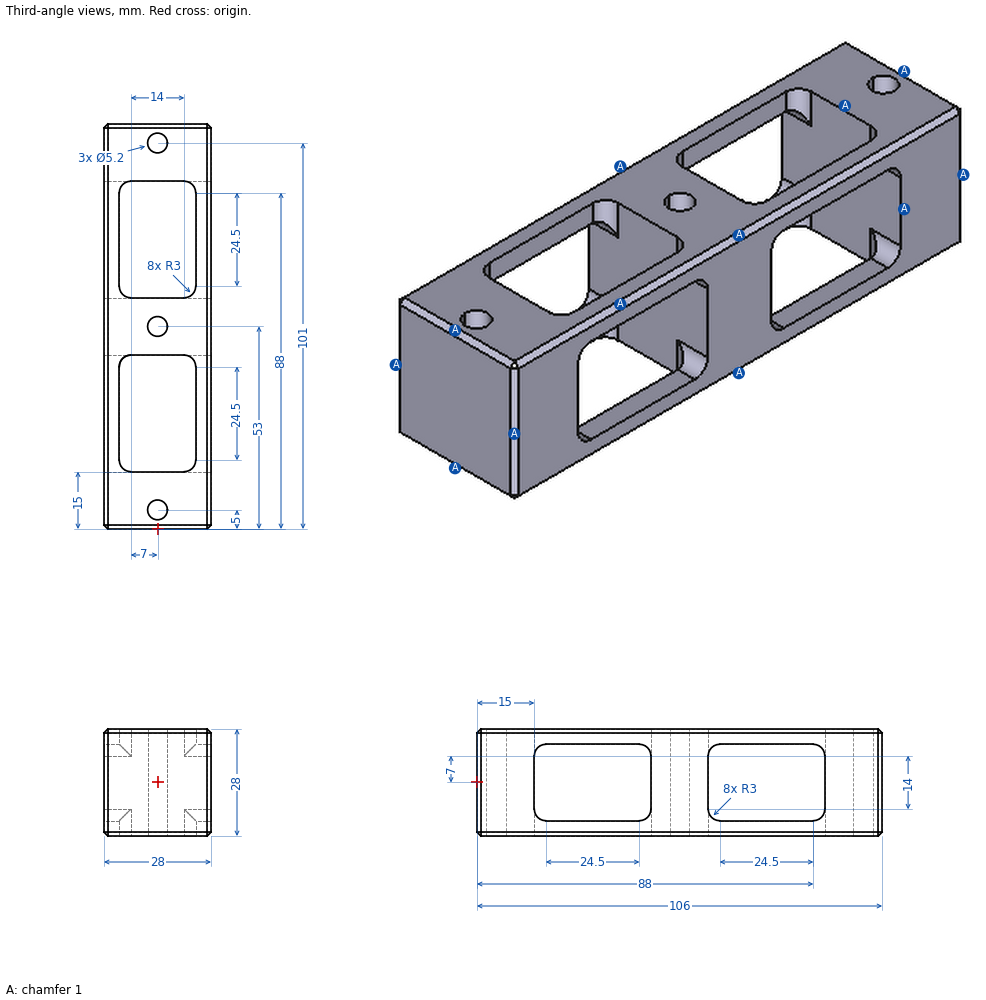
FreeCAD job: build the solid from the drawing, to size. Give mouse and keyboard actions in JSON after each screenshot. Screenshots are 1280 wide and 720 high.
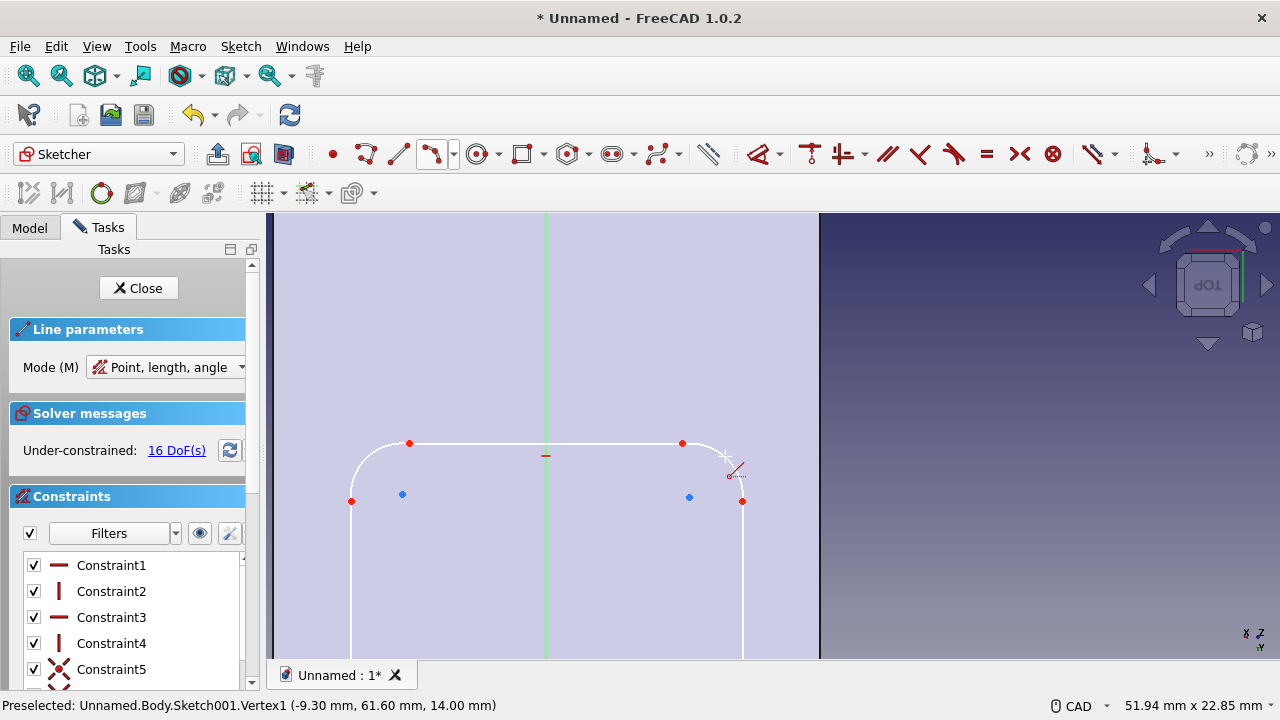
{"action": "scroll", "coordinate": [729, 462], "scroll_direction": "down", "scroll_amount": 10}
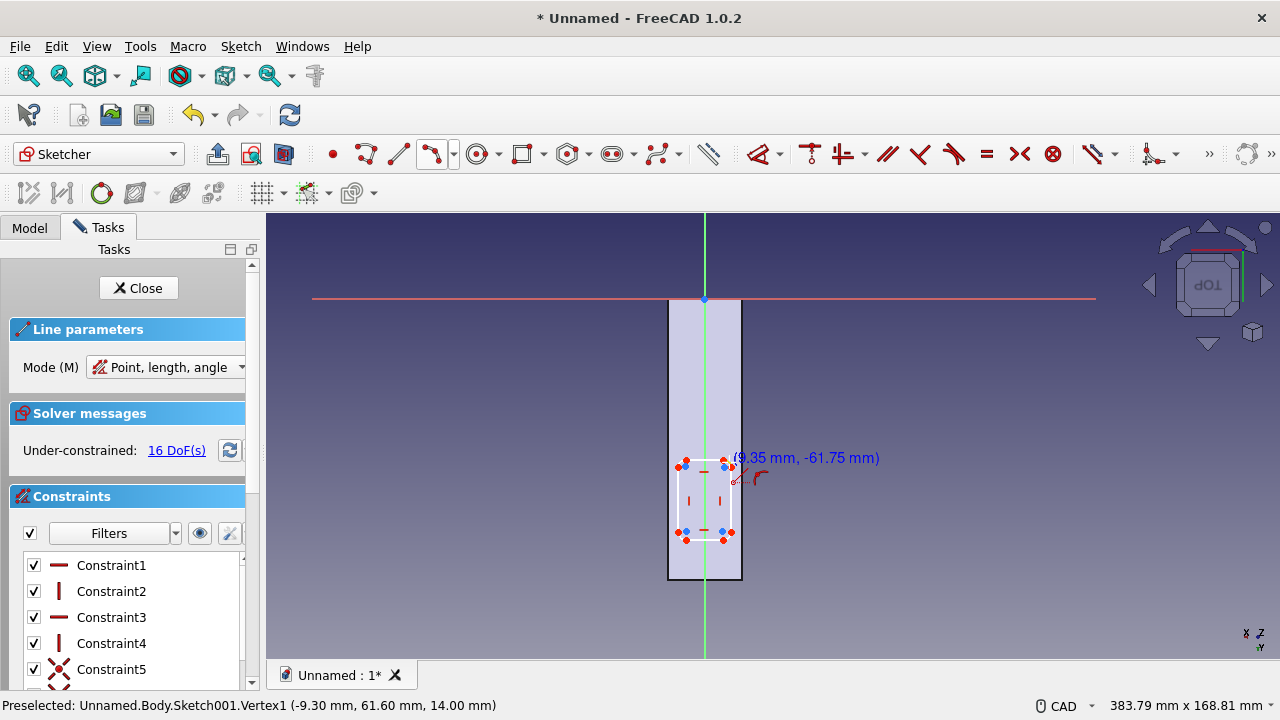
{"action": "left_click", "coordinate": [723, 339]}
{"action": "left_click", "coordinate": [686, 339]}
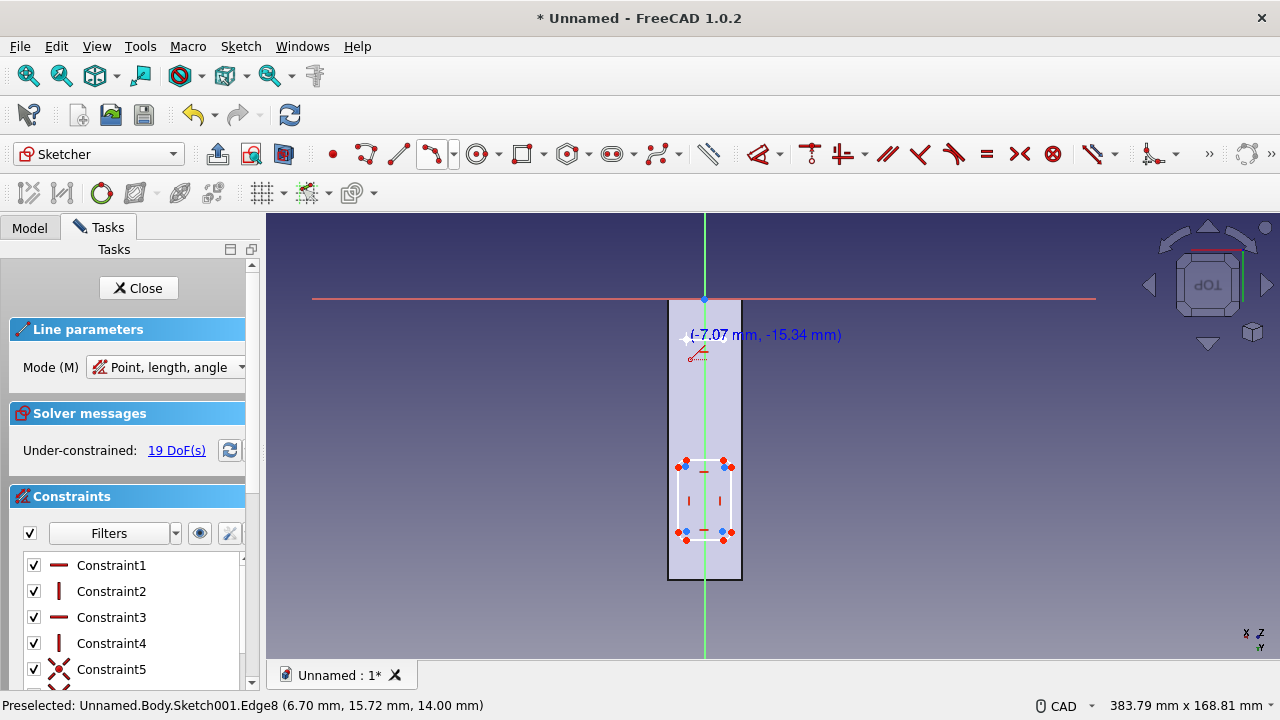
{"action": "scroll", "coordinate": [678, 347], "scroll_direction": "up", "scroll_amount": 2}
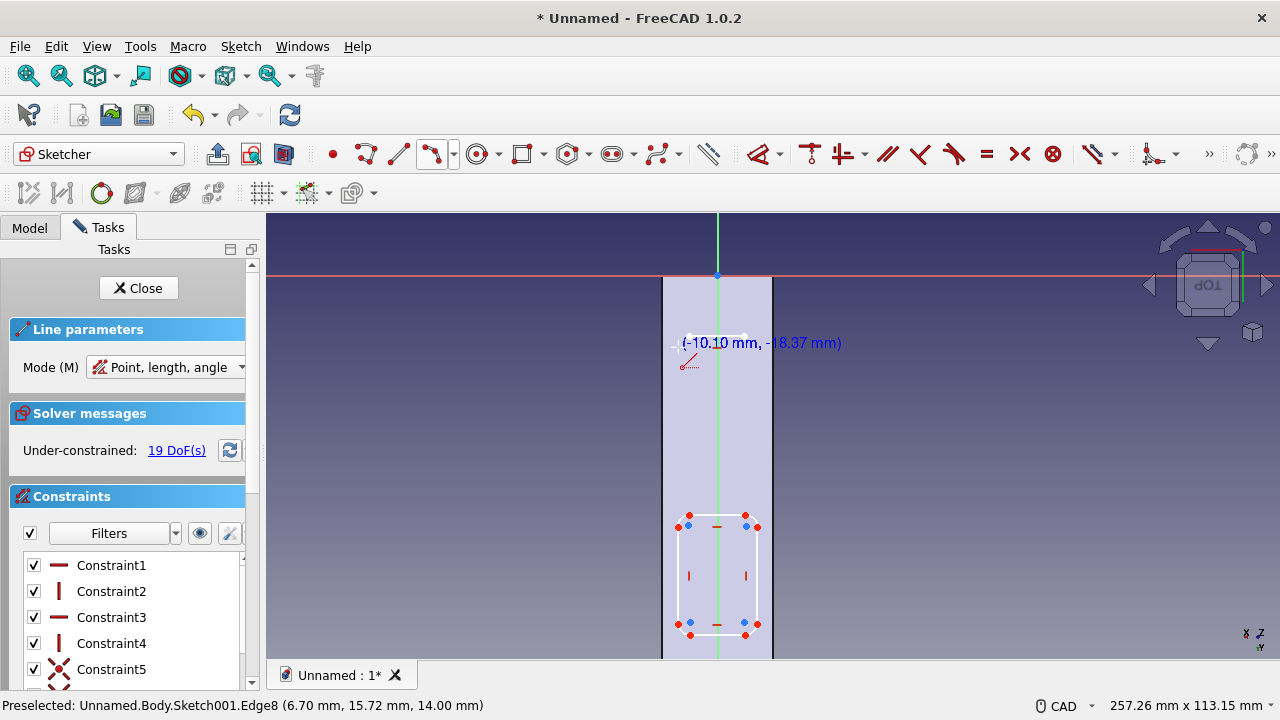
{"action": "left_click", "coordinate": [678, 347]}
{"action": "left_click", "coordinate": [678, 443]}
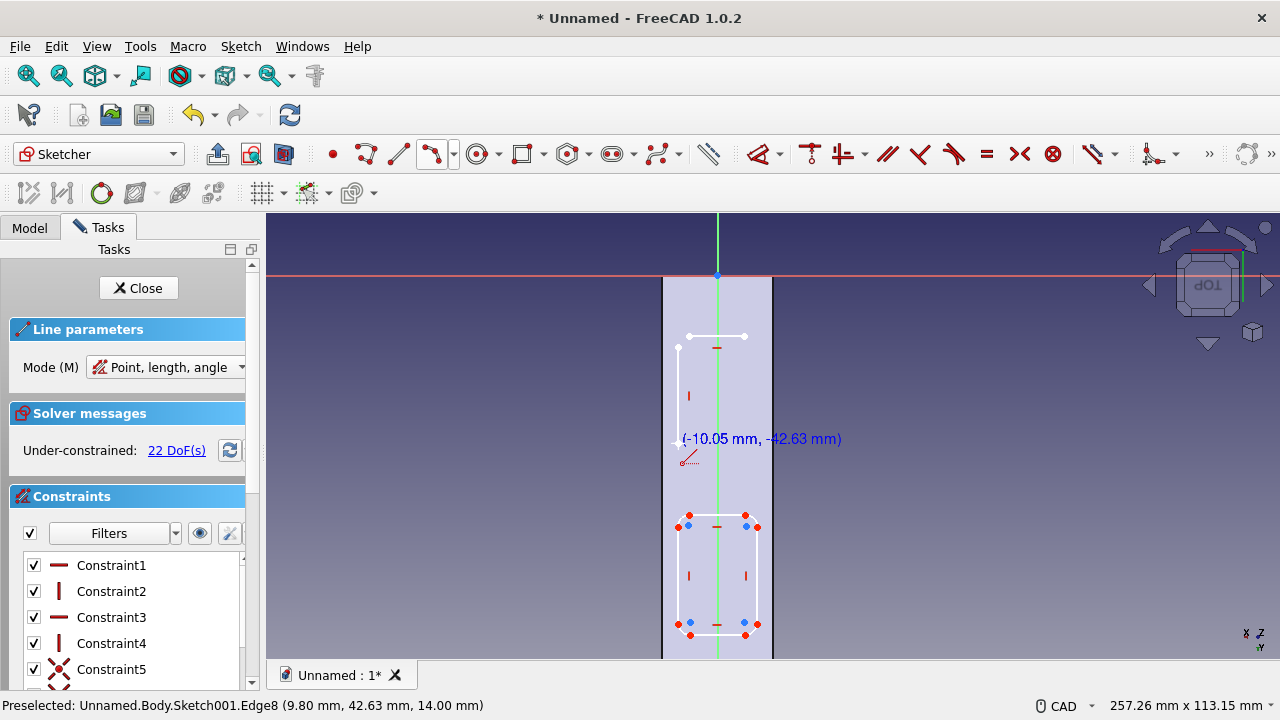
{"action": "left_click", "coordinate": [690, 455]}
{"action": "left_click", "coordinate": [745, 455]}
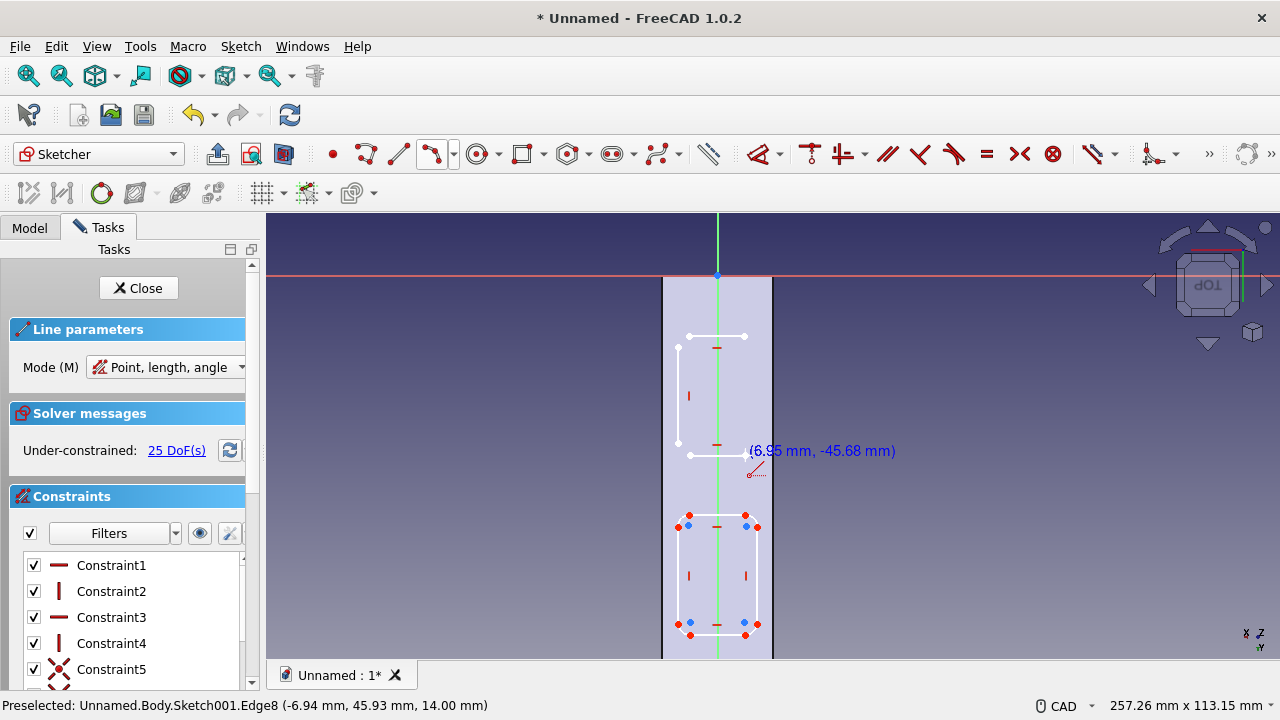
{"action": "left_click", "coordinate": [757, 443]}
{"action": "left_click", "coordinate": [757, 347]}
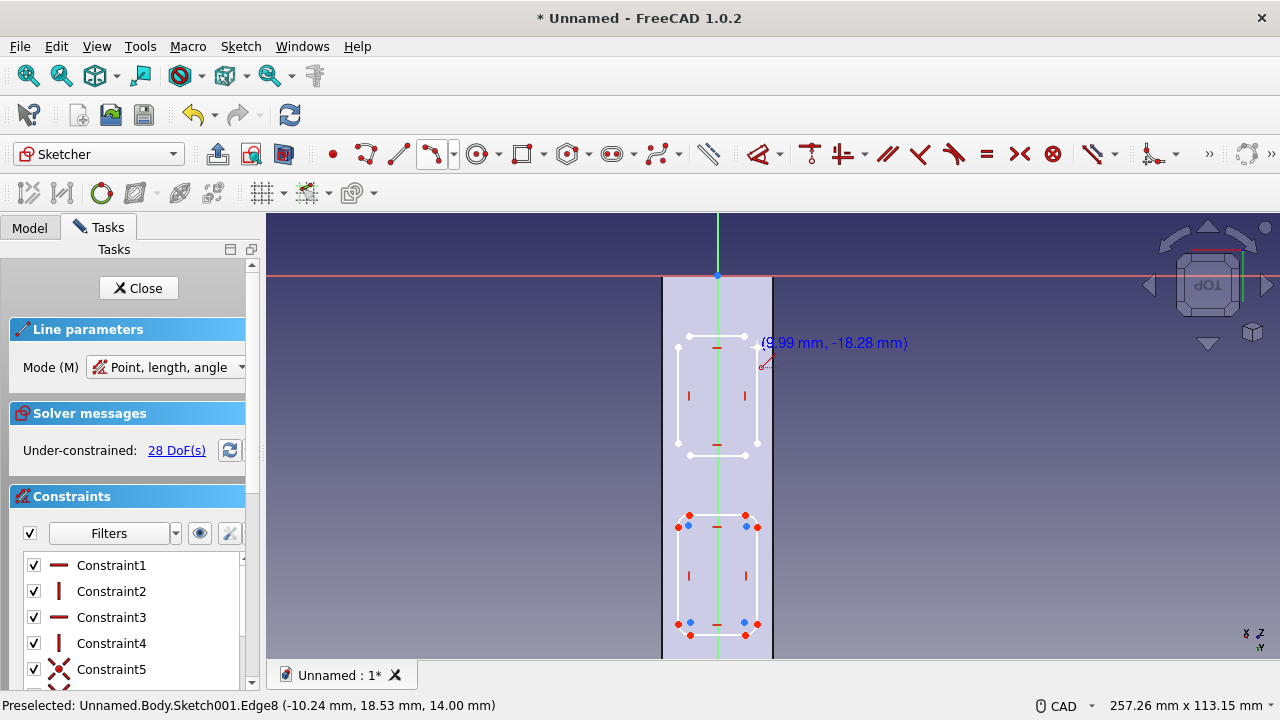
{"action": "left_click", "coordinate": [432, 154]}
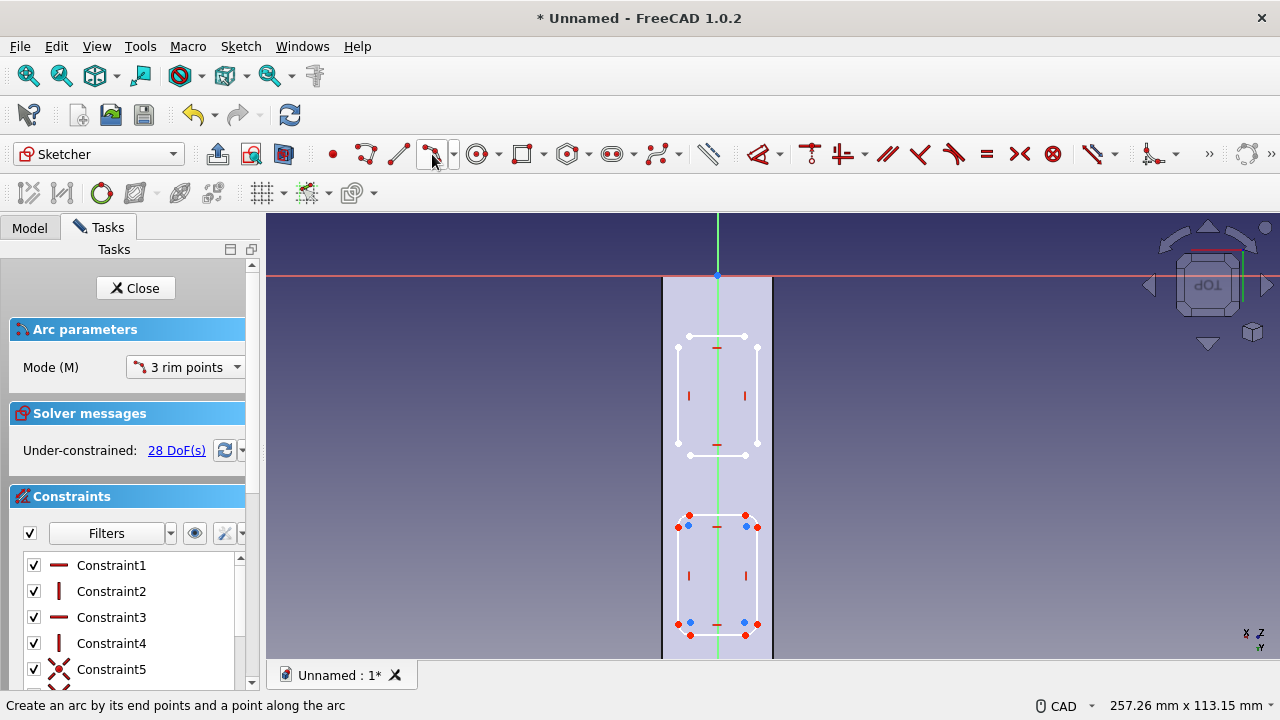
{"action": "left_click", "coordinate": [690, 336]}
{"action": "left_click", "coordinate": [678, 348]}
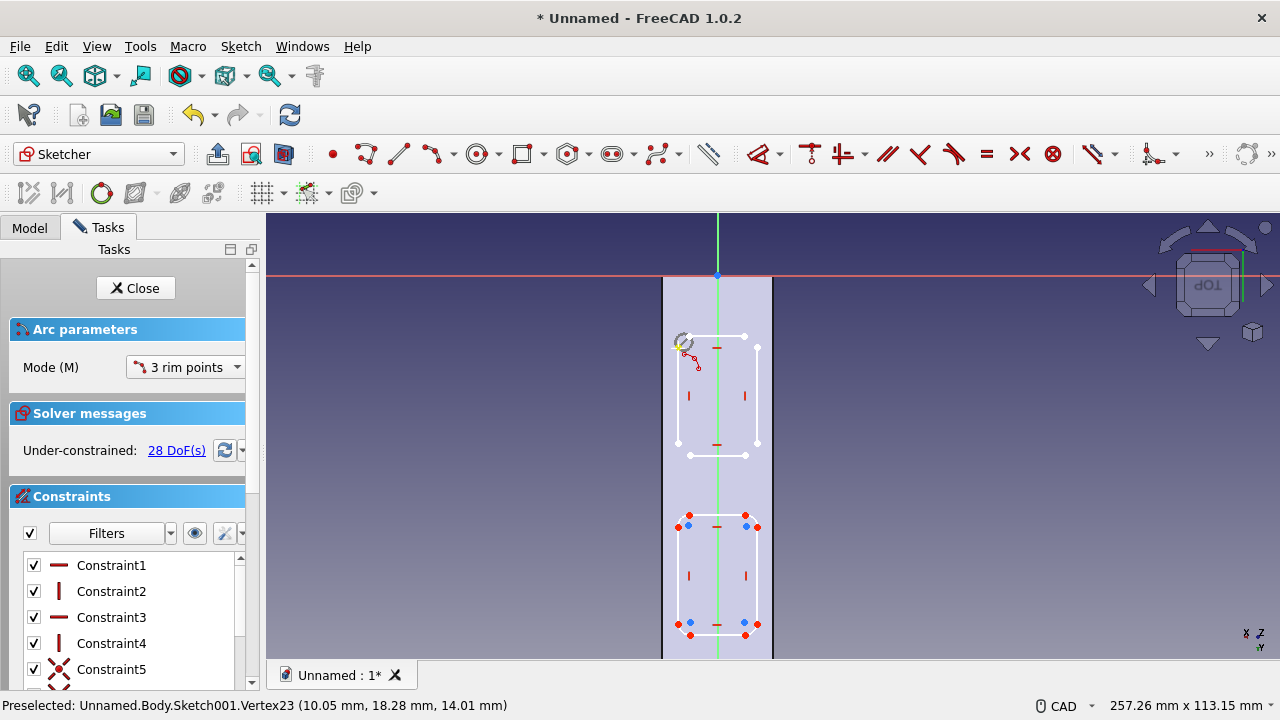
{"action": "scroll", "coordinate": [682, 339], "scroll_direction": "up", "scroll_amount": 8}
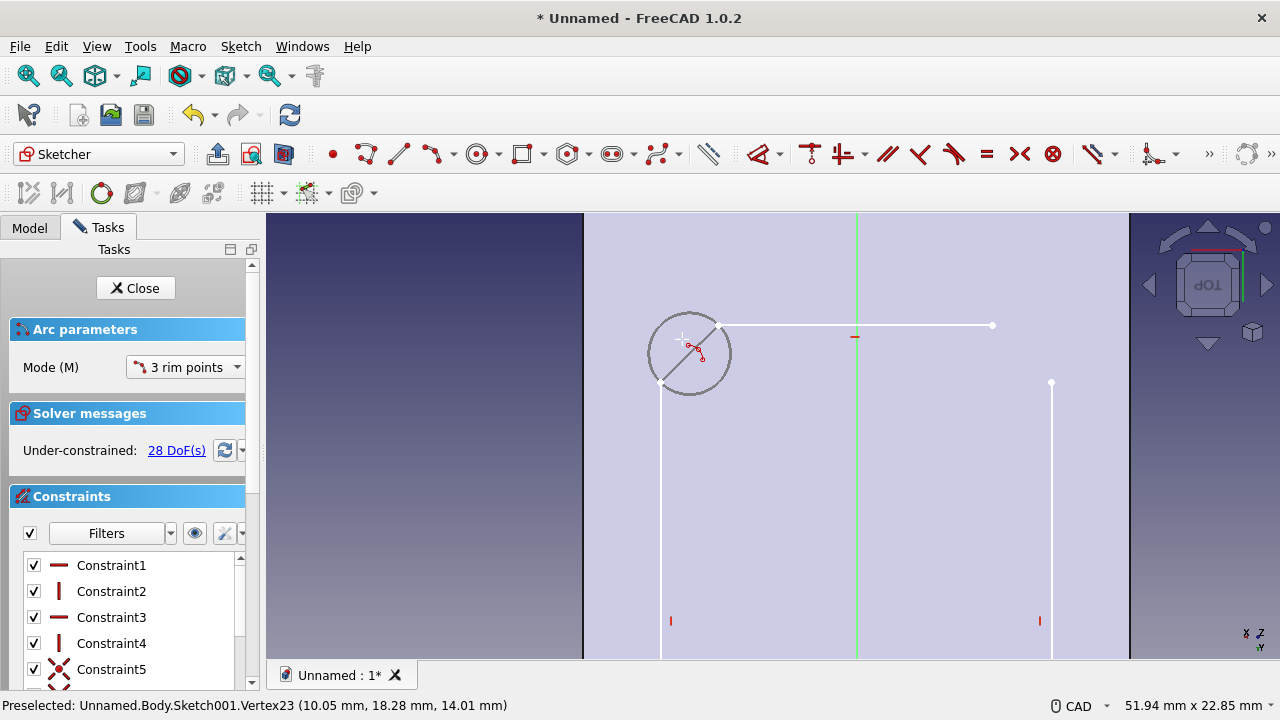
{"action": "left_click", "coordinate": [679, 336]}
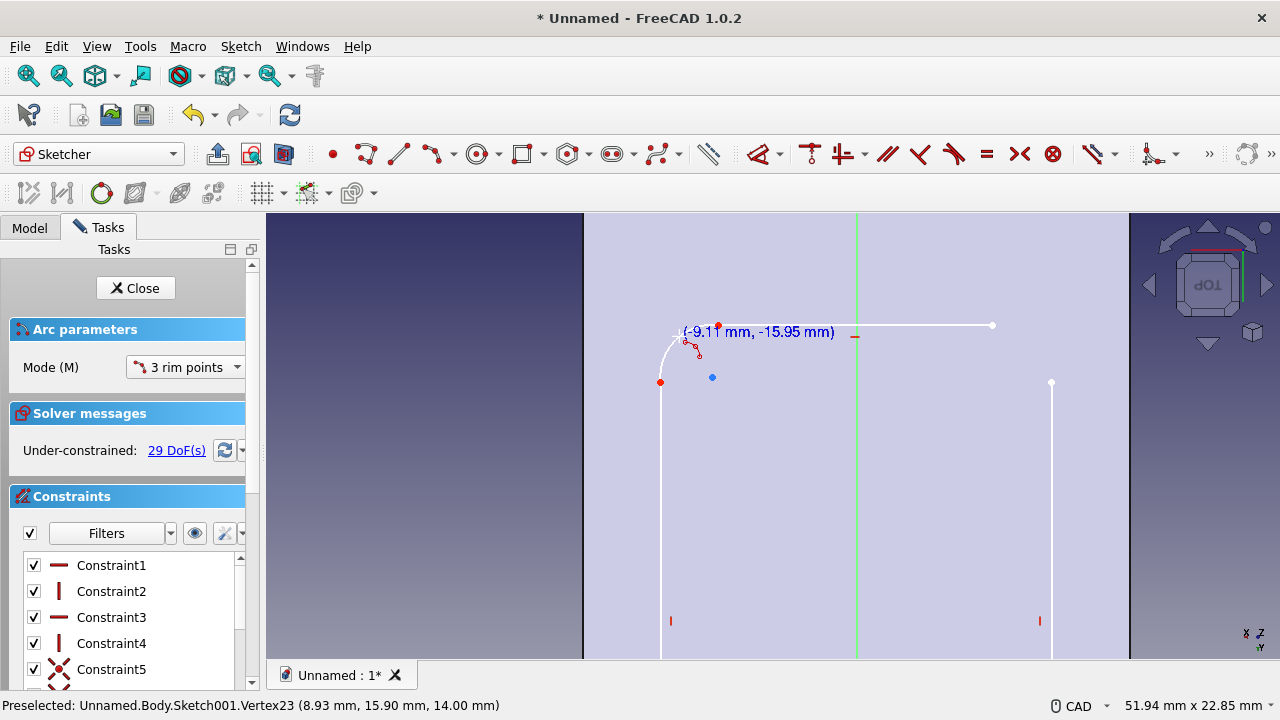
{"action": "scroll", "coordinate": [681, 342], "scroll_direction": "down", "scroll_amount": 10}